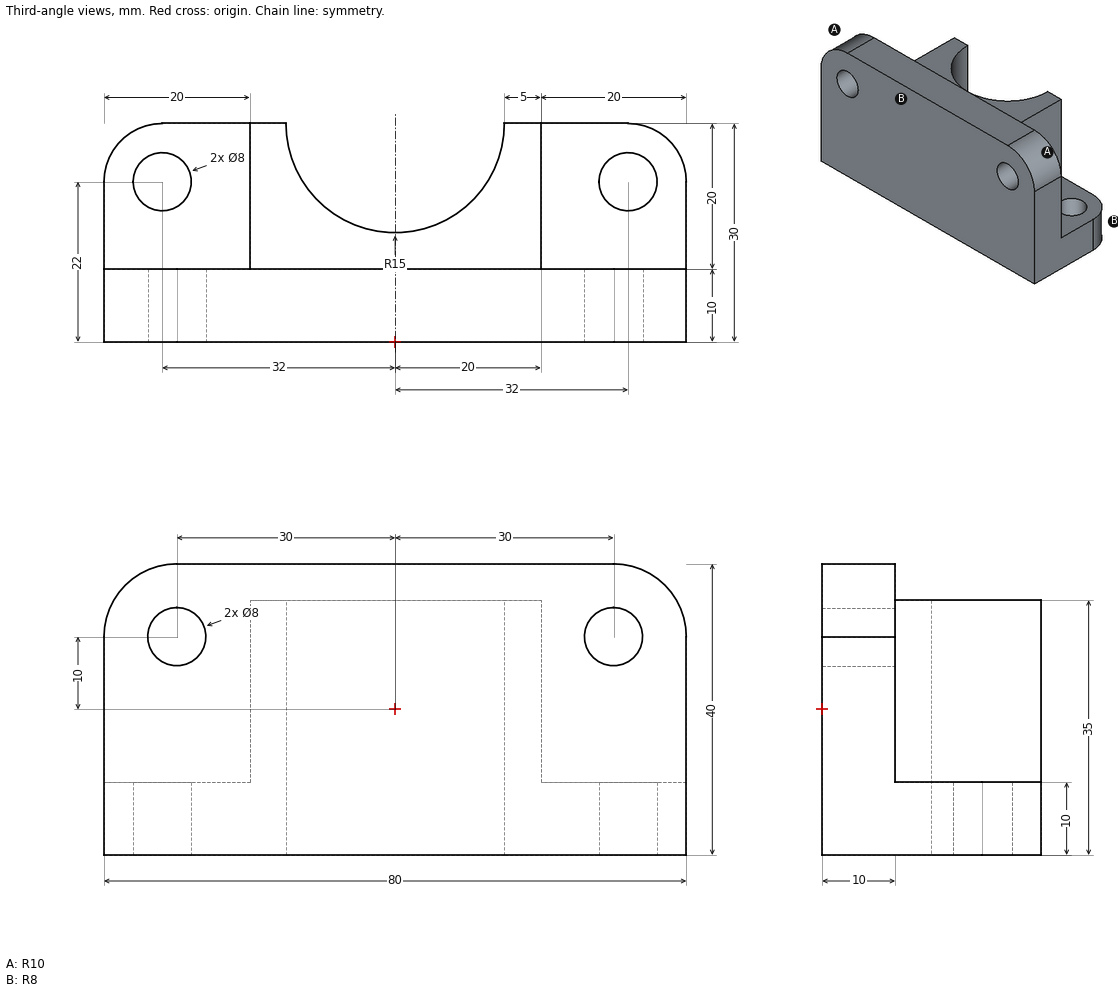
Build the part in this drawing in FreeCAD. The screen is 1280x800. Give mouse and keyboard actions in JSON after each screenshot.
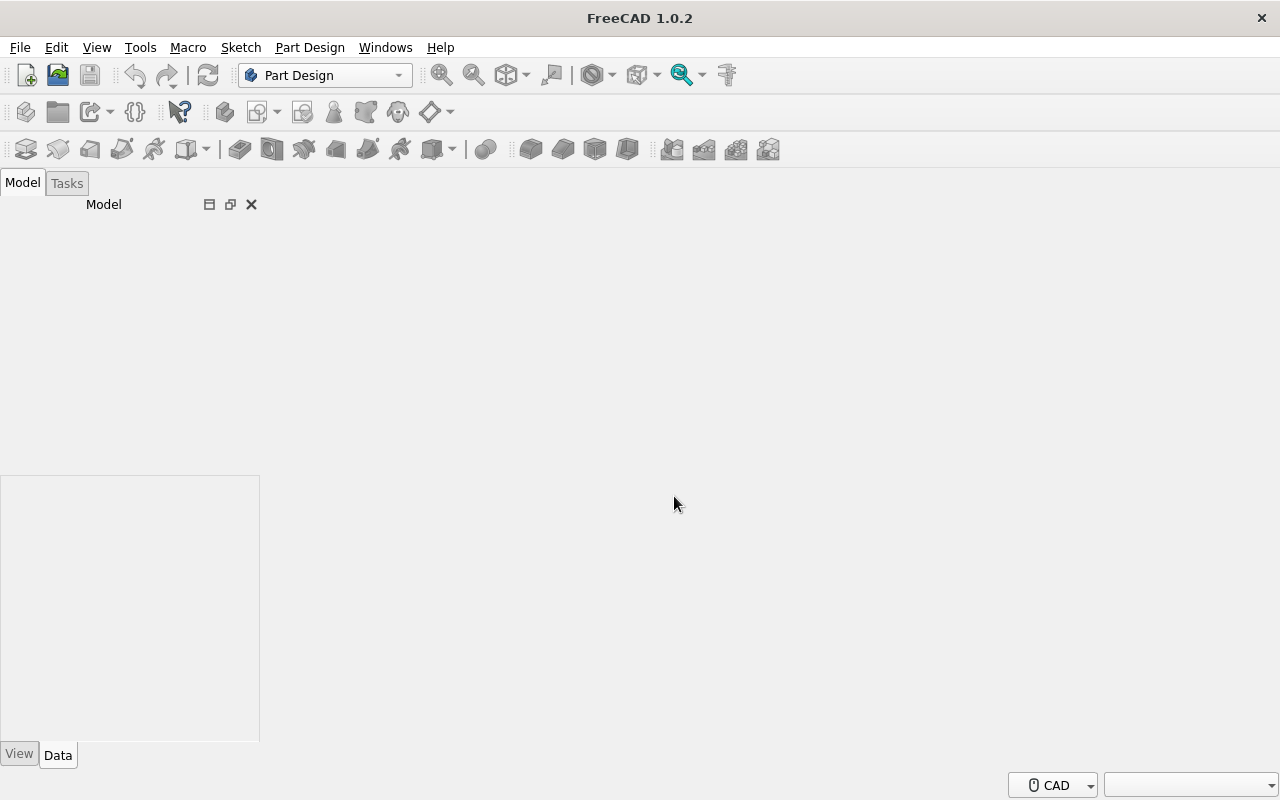
{"action": "left_click", "coordinate": [26, 76]}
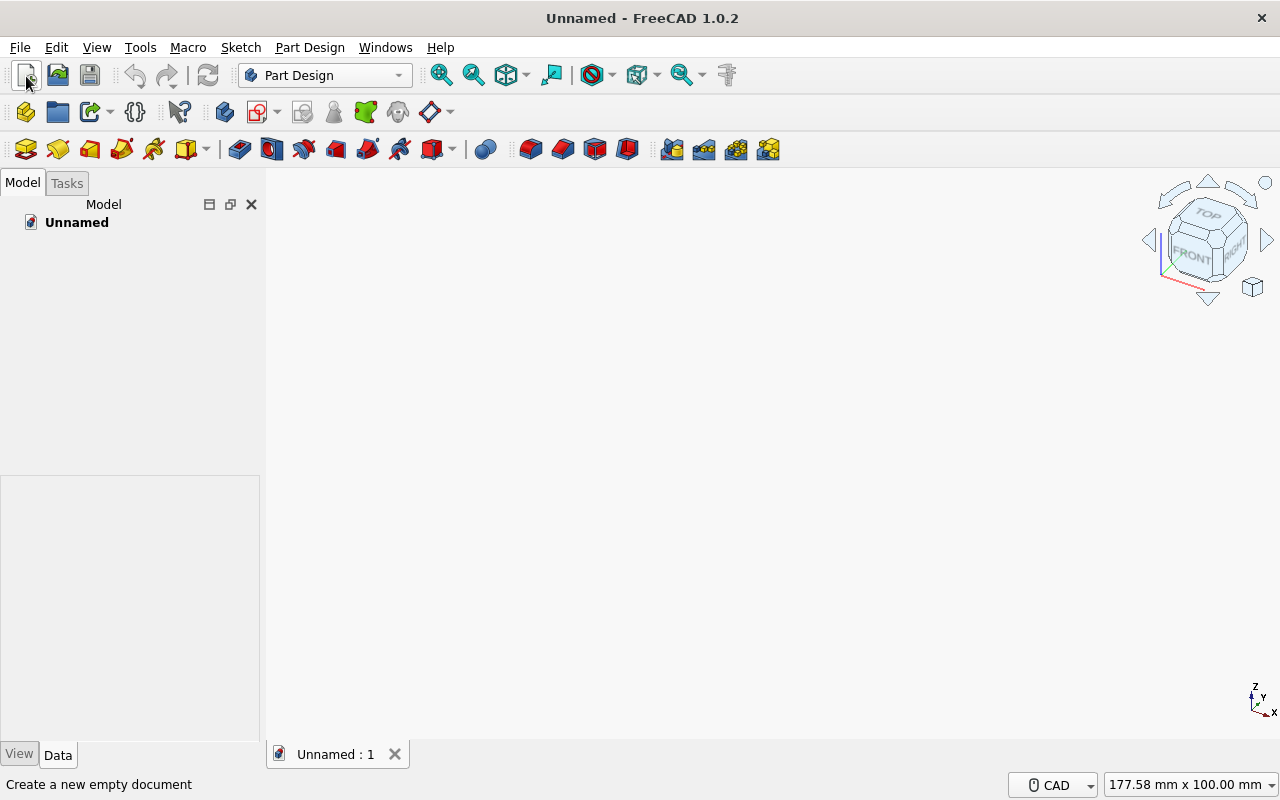
{"action": "left_click", "coordinate": [258, 112]}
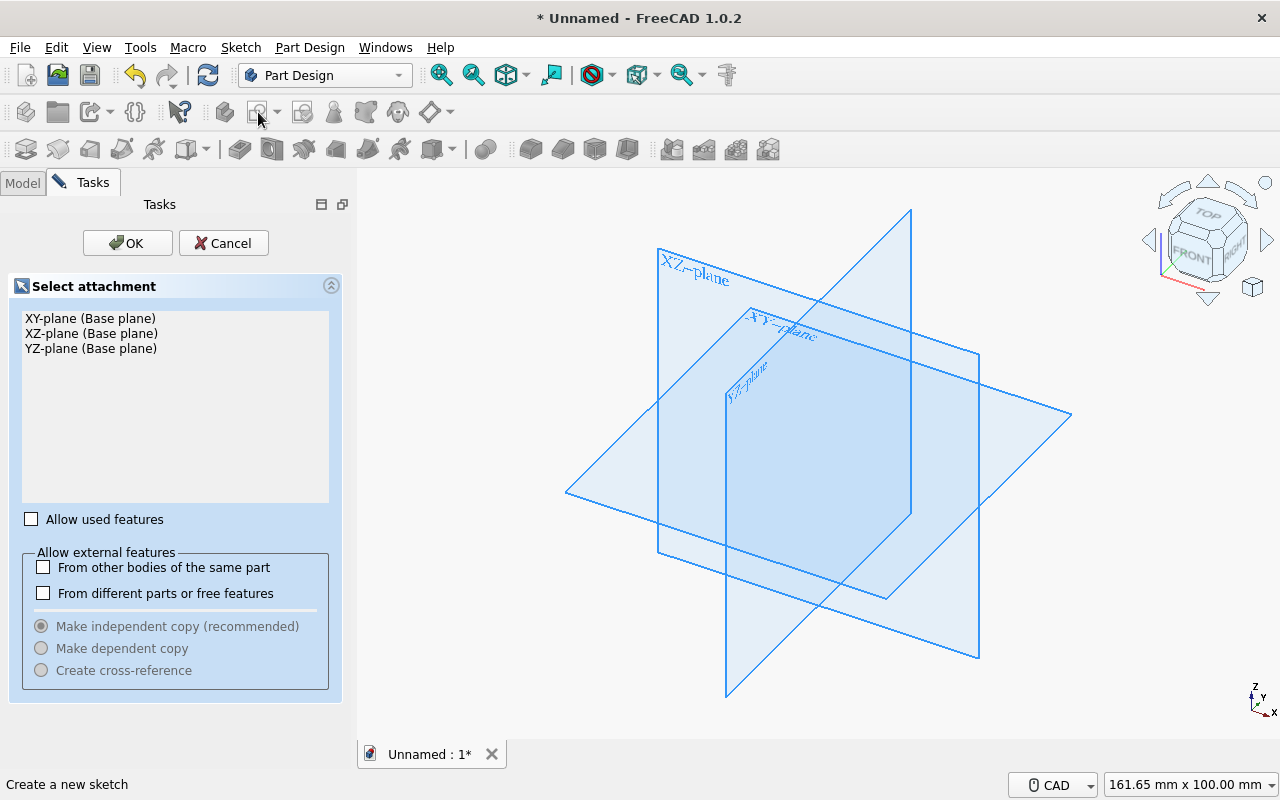
{"action": "left_click", "coordinate": [82, 334]}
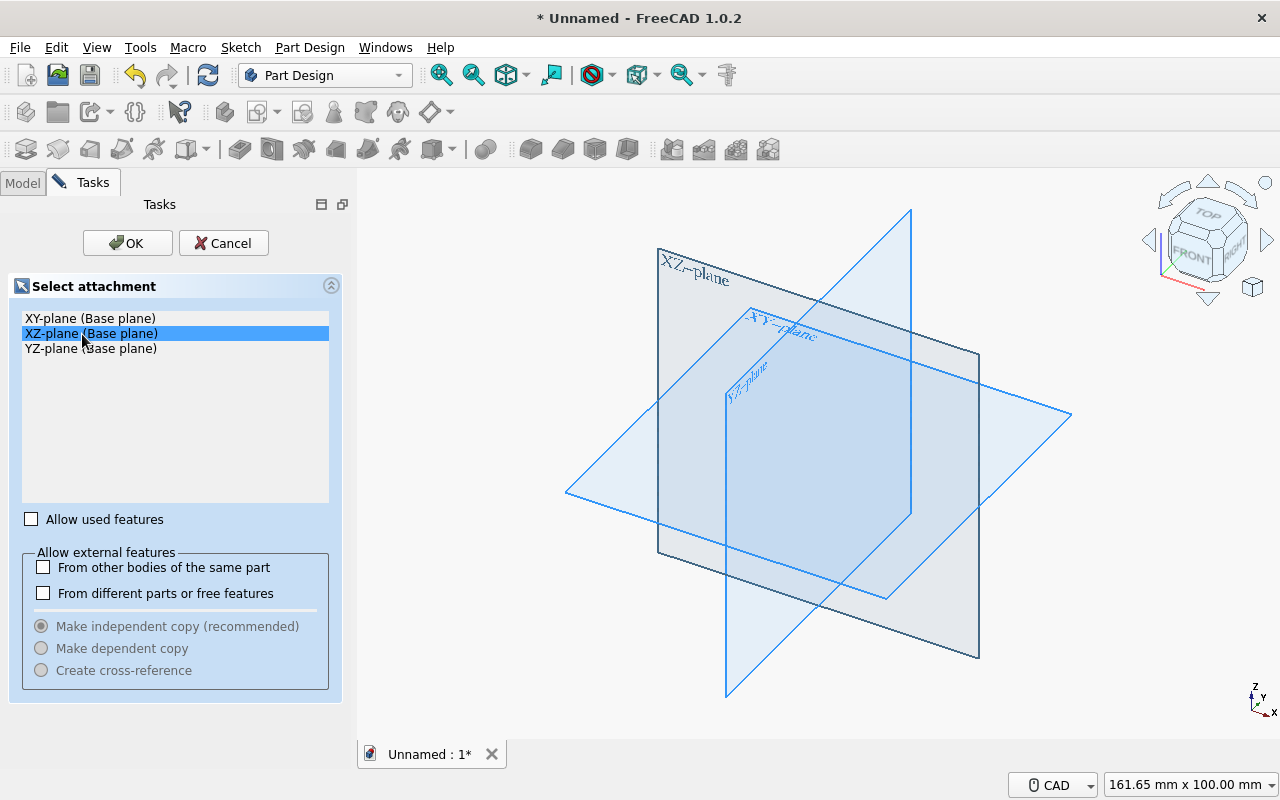
{"action": "left_click", "coordinate": [128, 243]}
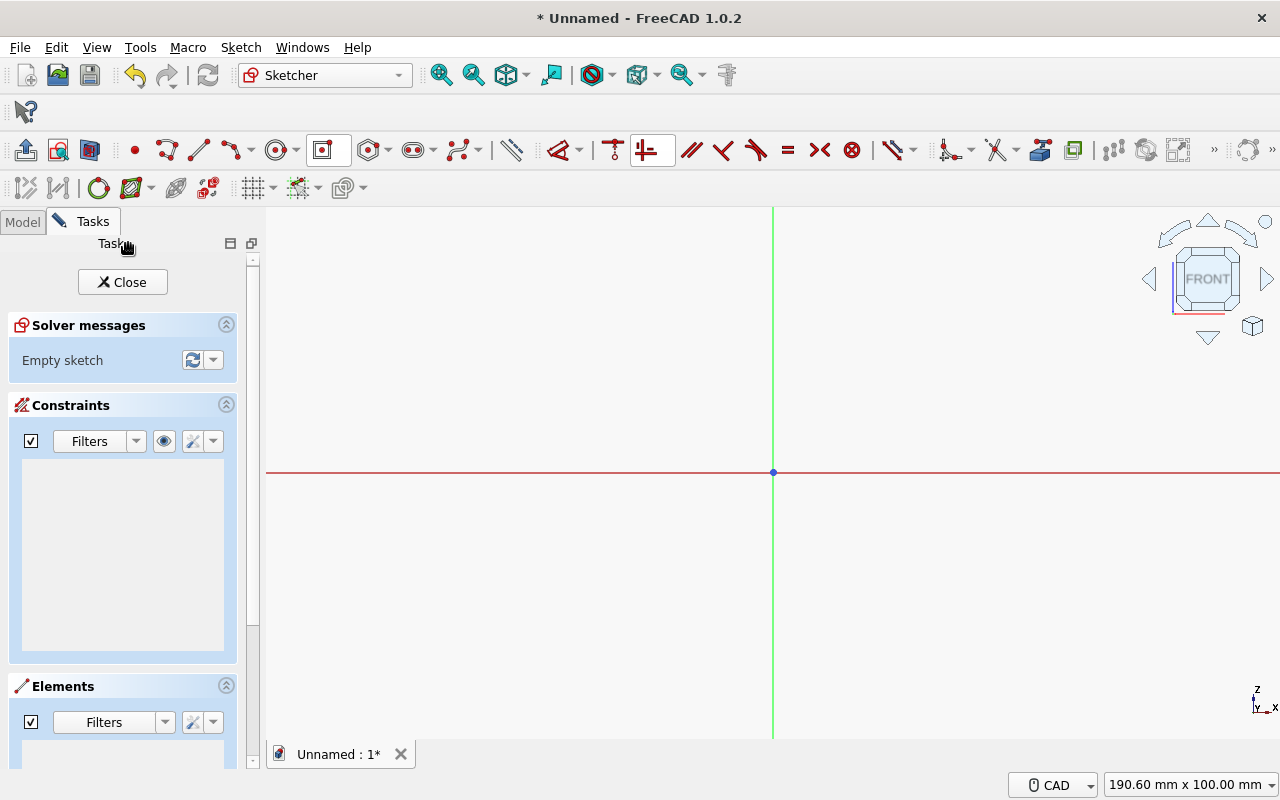
{"action": "scroll", "coordinate": [912, 473], "scroll_direction": "up", "scroll_amount": 2}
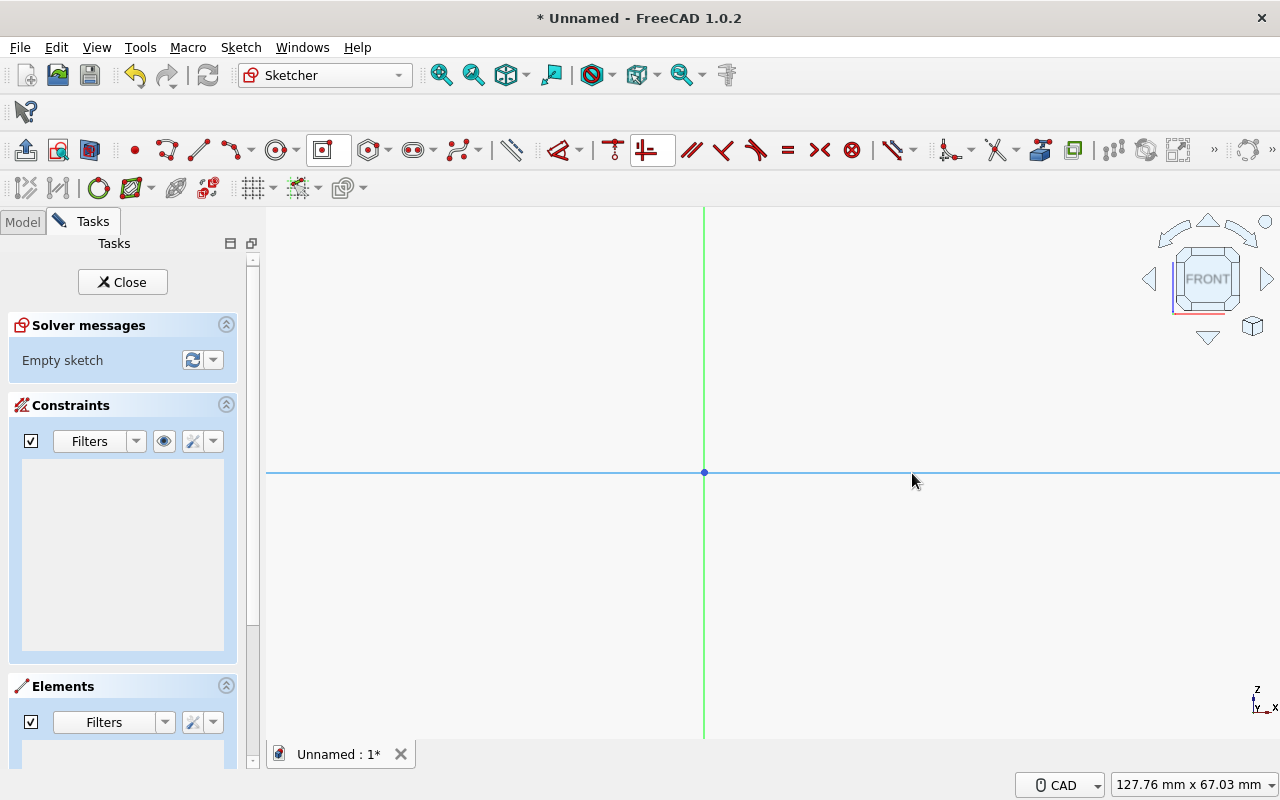
{"action": "left_click", "coordinate": [322, 150]}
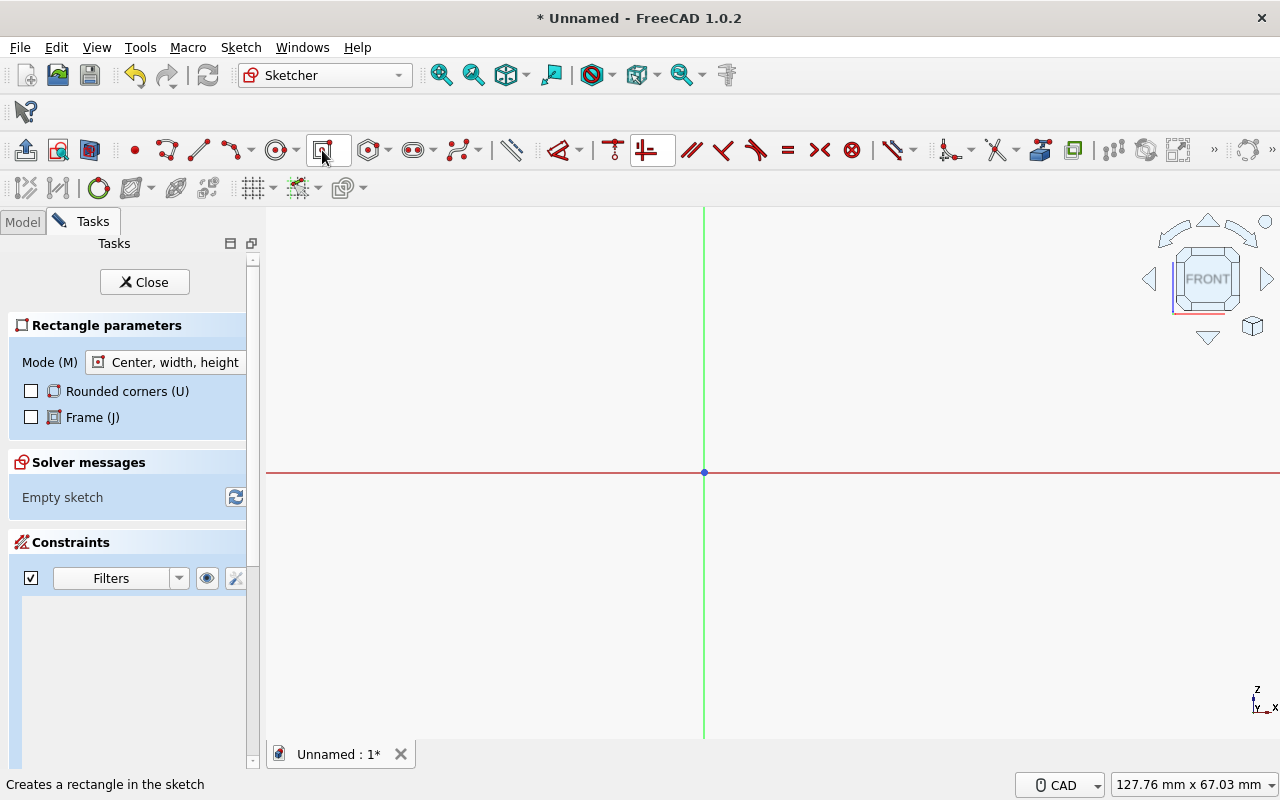
{"action": "left_click", "coordinate": [704, 473]}
{"action": "mouse_move", "coordinate": [1022, 314]}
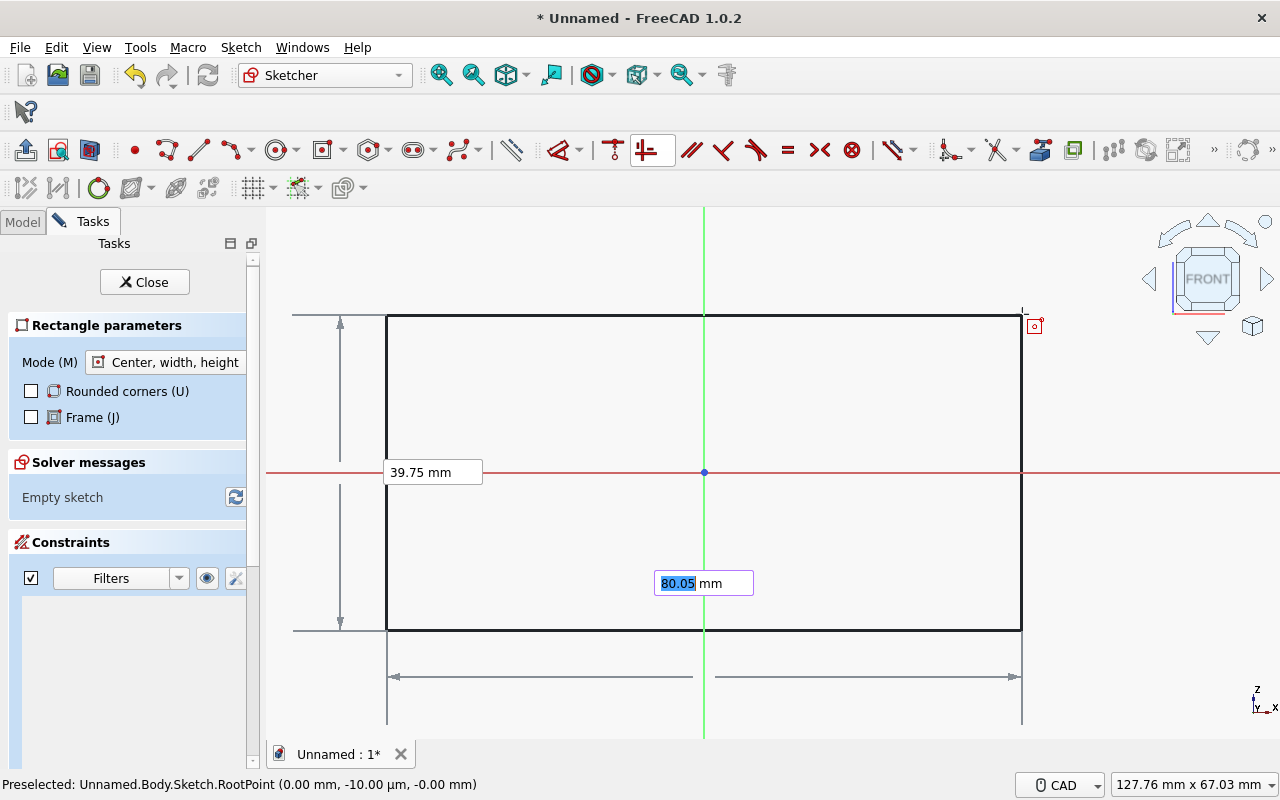
{"action": "type", "text": "80"}
{"action": "key", "text": "Tab"}
{"action": "type", "text": "40"}
{"action": "key", "text": "Return"}
{"action": "key", "text": "Escape"}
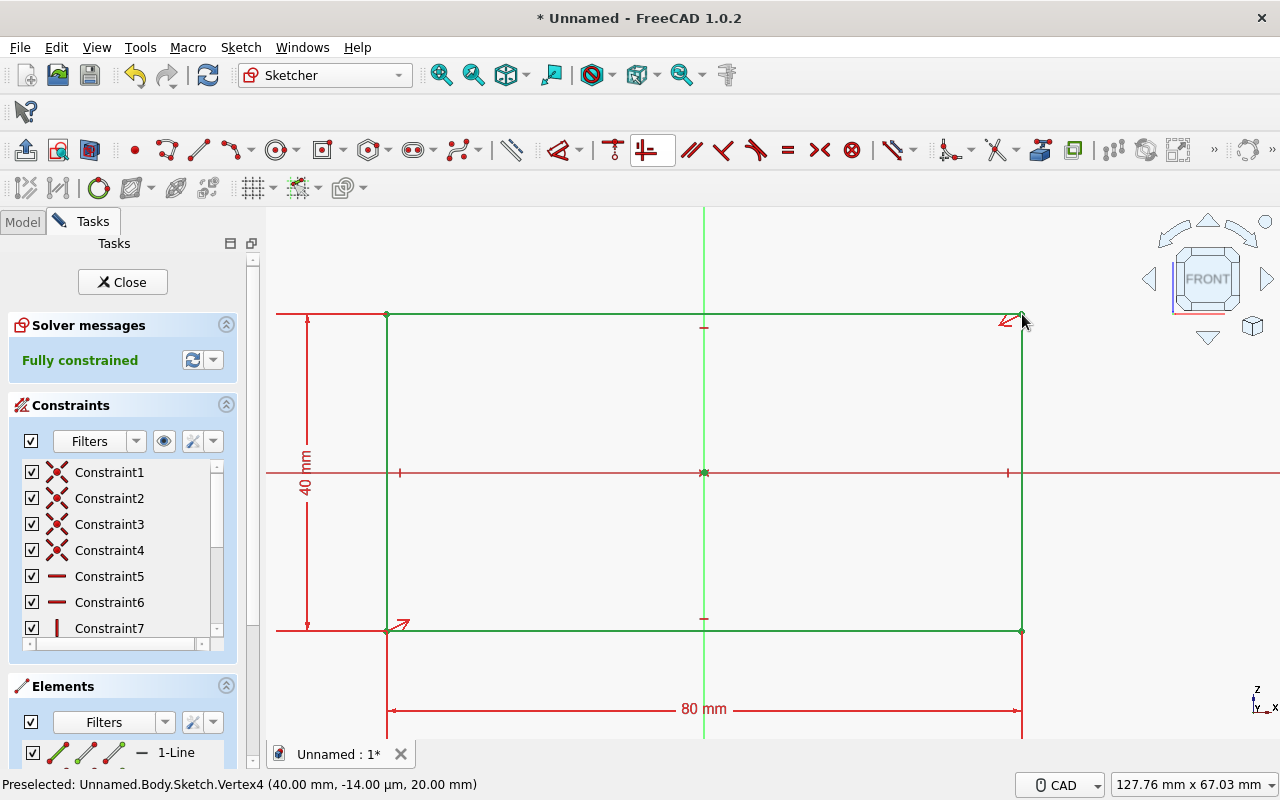
{"action": "left_click", "coordinate": [123, 282]}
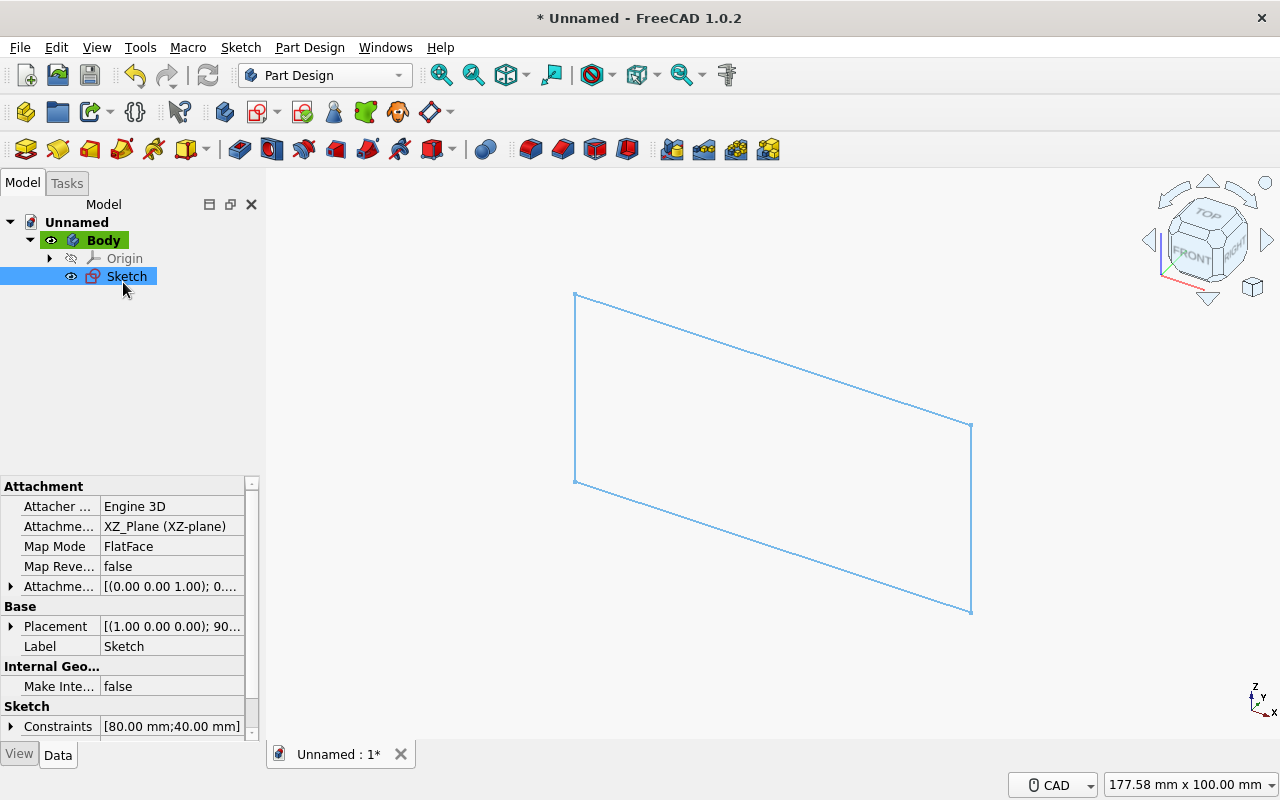
{"action": "left_click", "coordinate": [26, 150]}